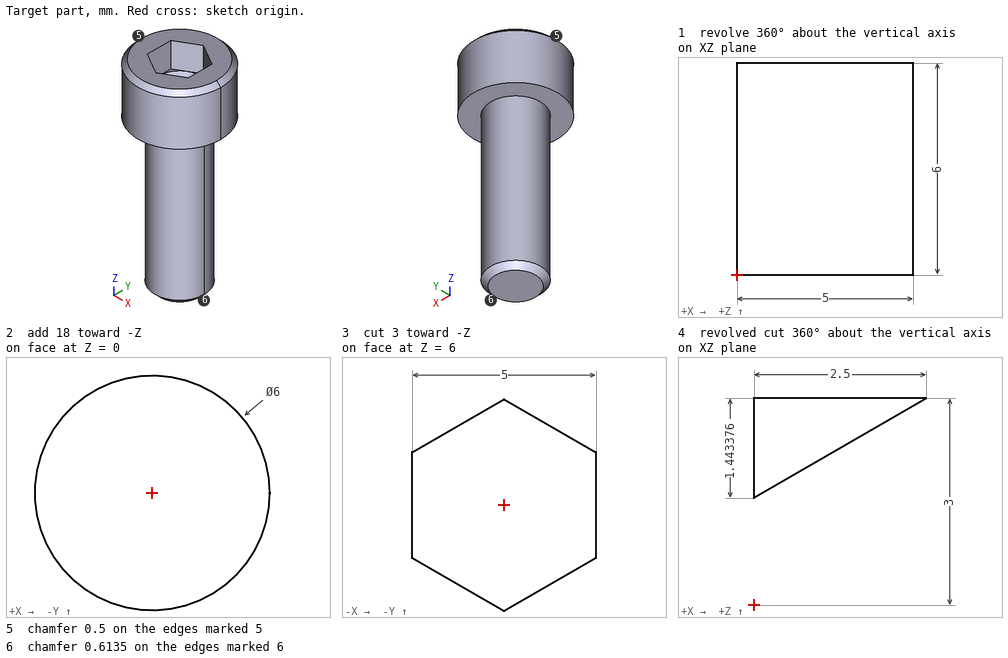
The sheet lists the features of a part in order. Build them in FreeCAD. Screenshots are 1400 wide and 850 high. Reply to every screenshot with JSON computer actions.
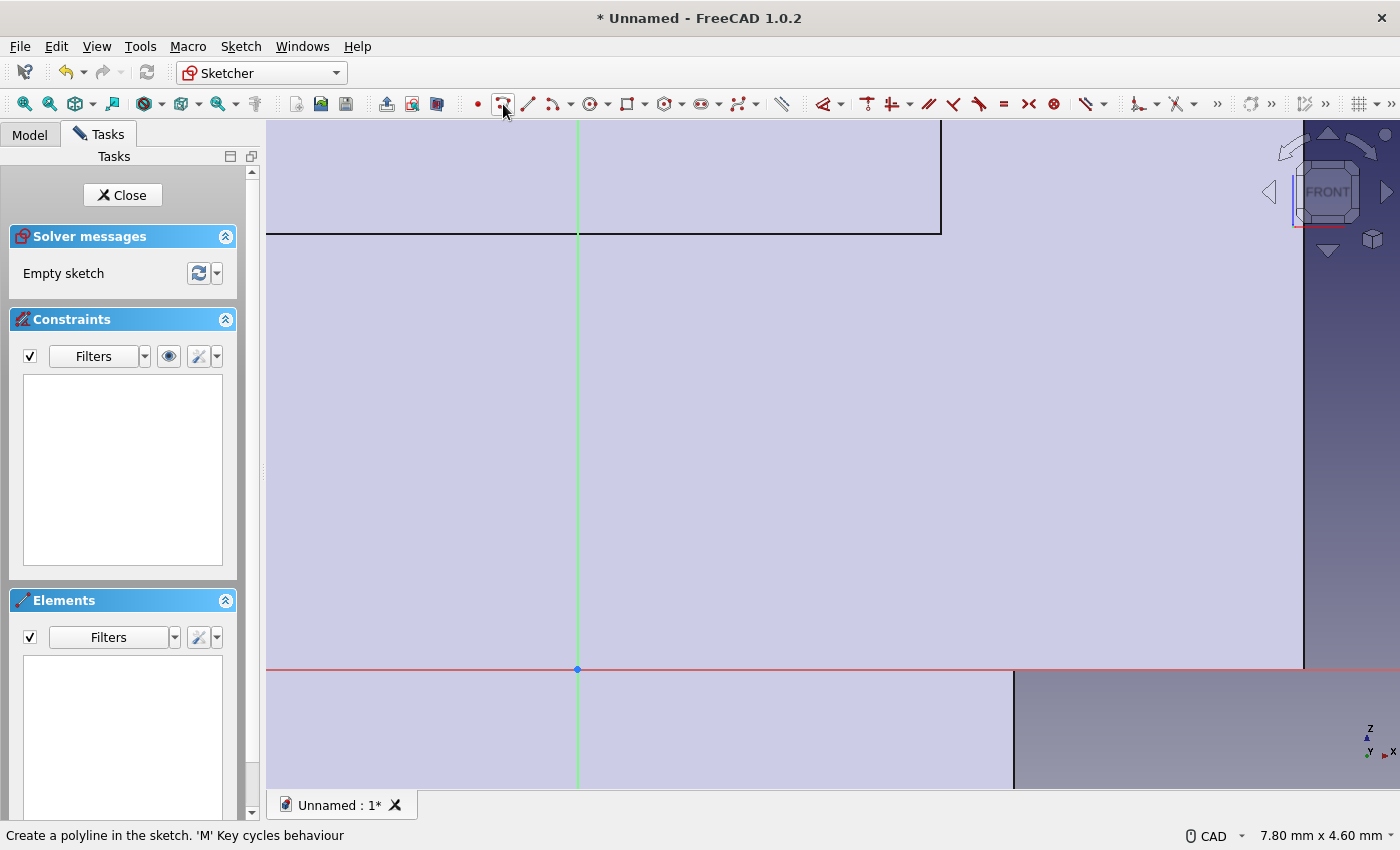
{"action": "left_click", "coordinate": [578, 444]}
{"action": "left_click", "coordinate": [941, 234]}
{"action": "left_click", "coordinate": [587, 234]}
{"action": "left_click", "coordinate": [578, 445]}
{"action": "key", "text": "Escape"}
{"action": "key", "text": "Escape"}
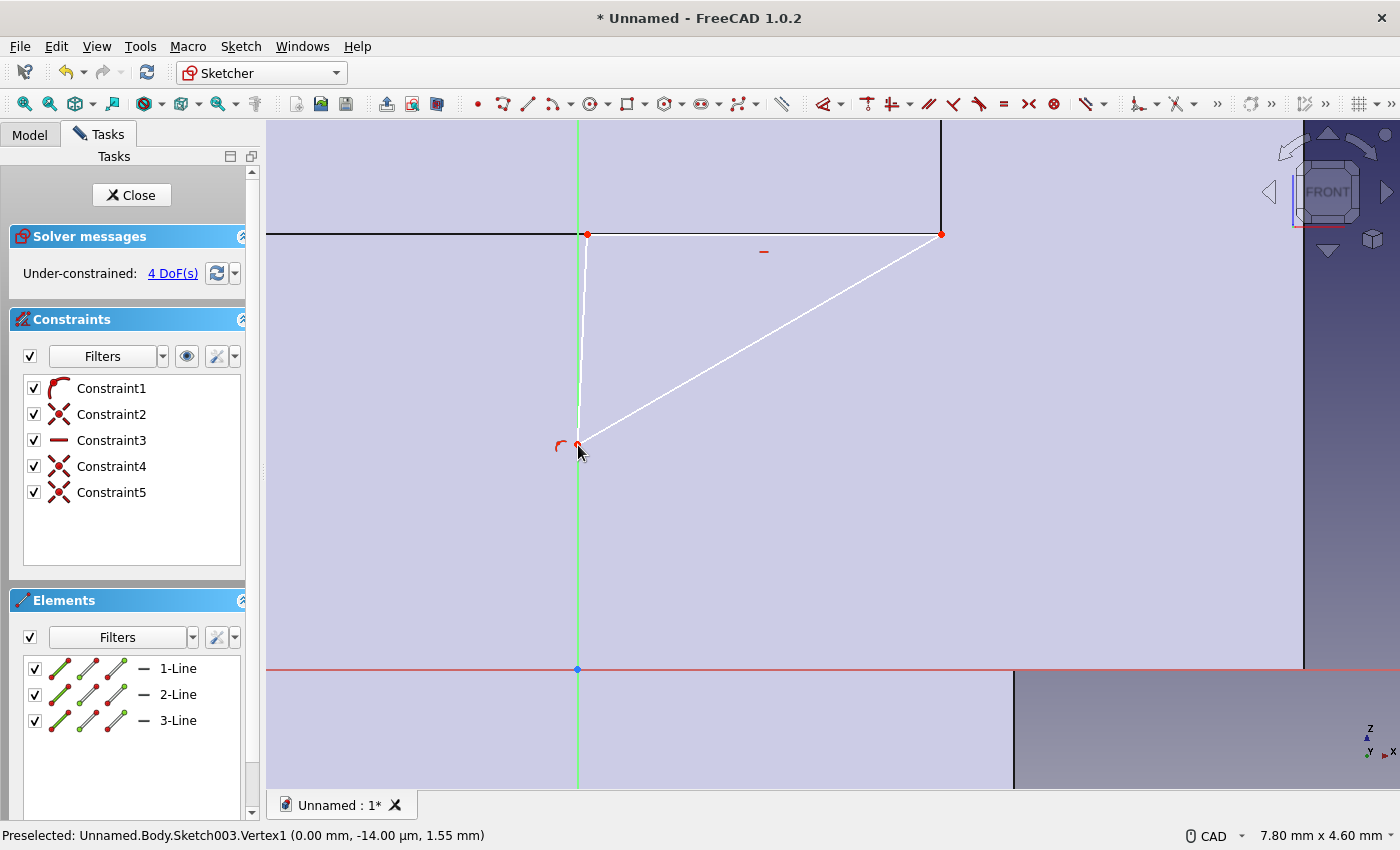
{"action": "left_click", "coordinate": [581, 382]}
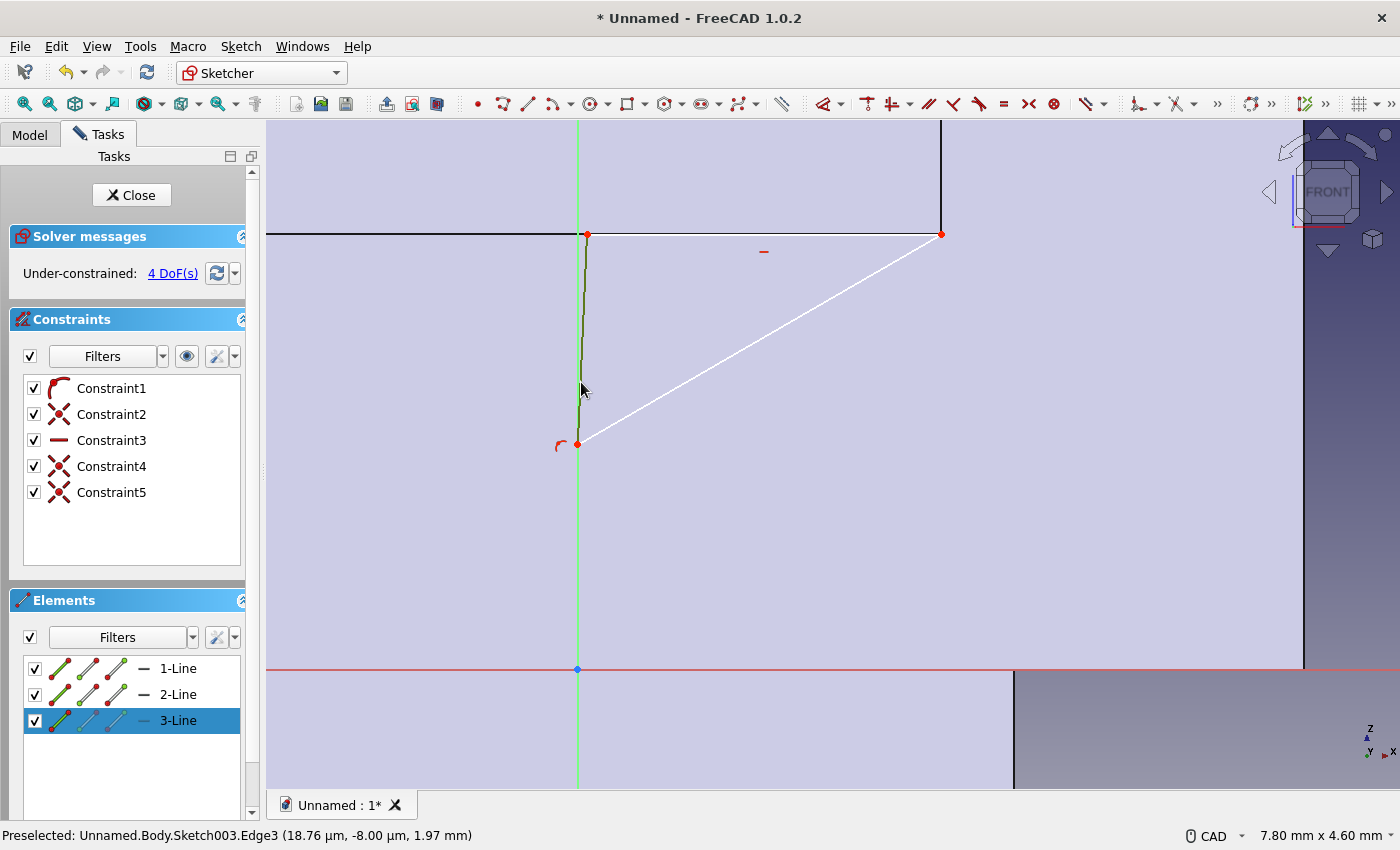
{"action": "left_click", "coordinate": [910, 104]}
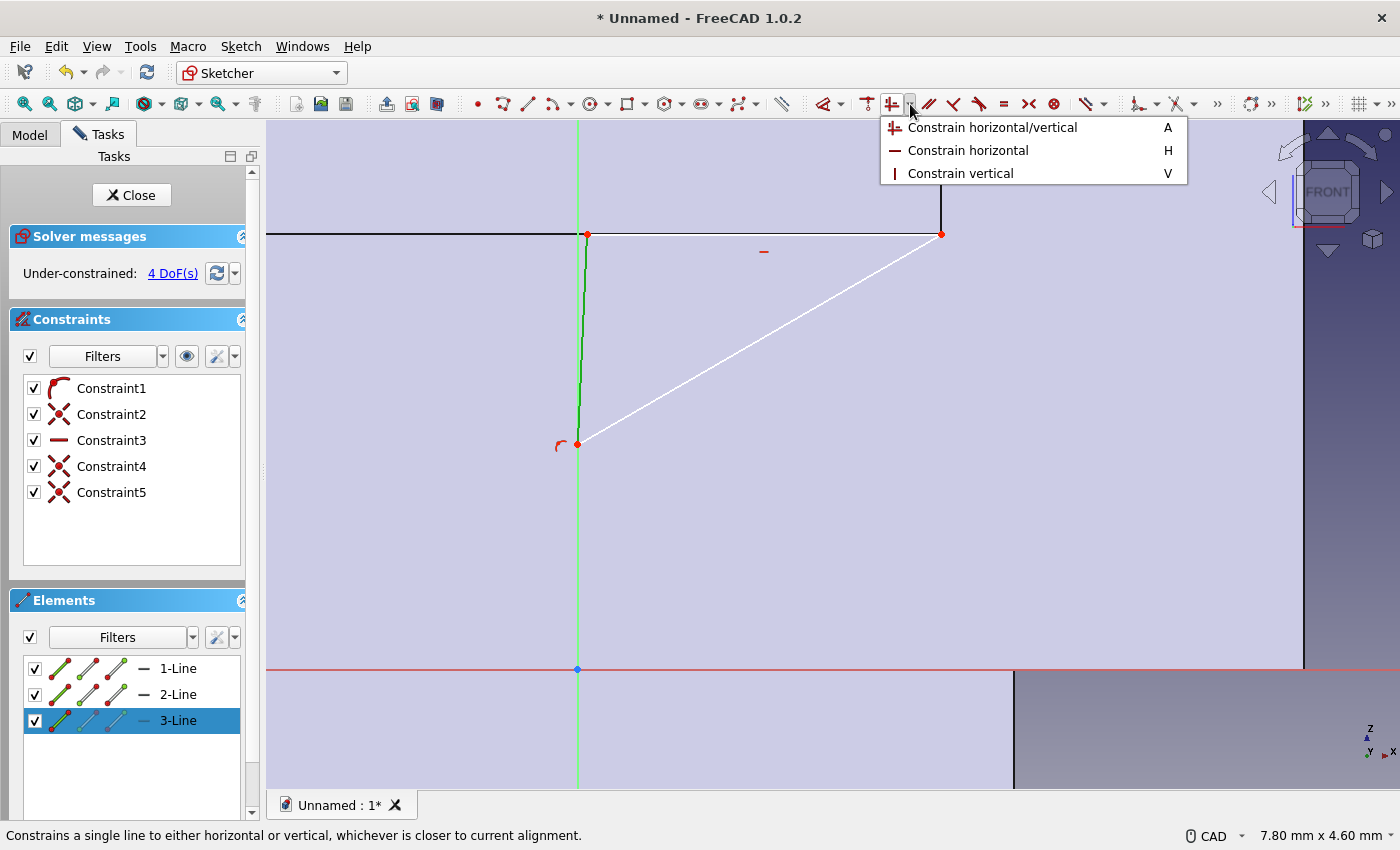
{"action": "left_click", "coordinate": [1034, 174]}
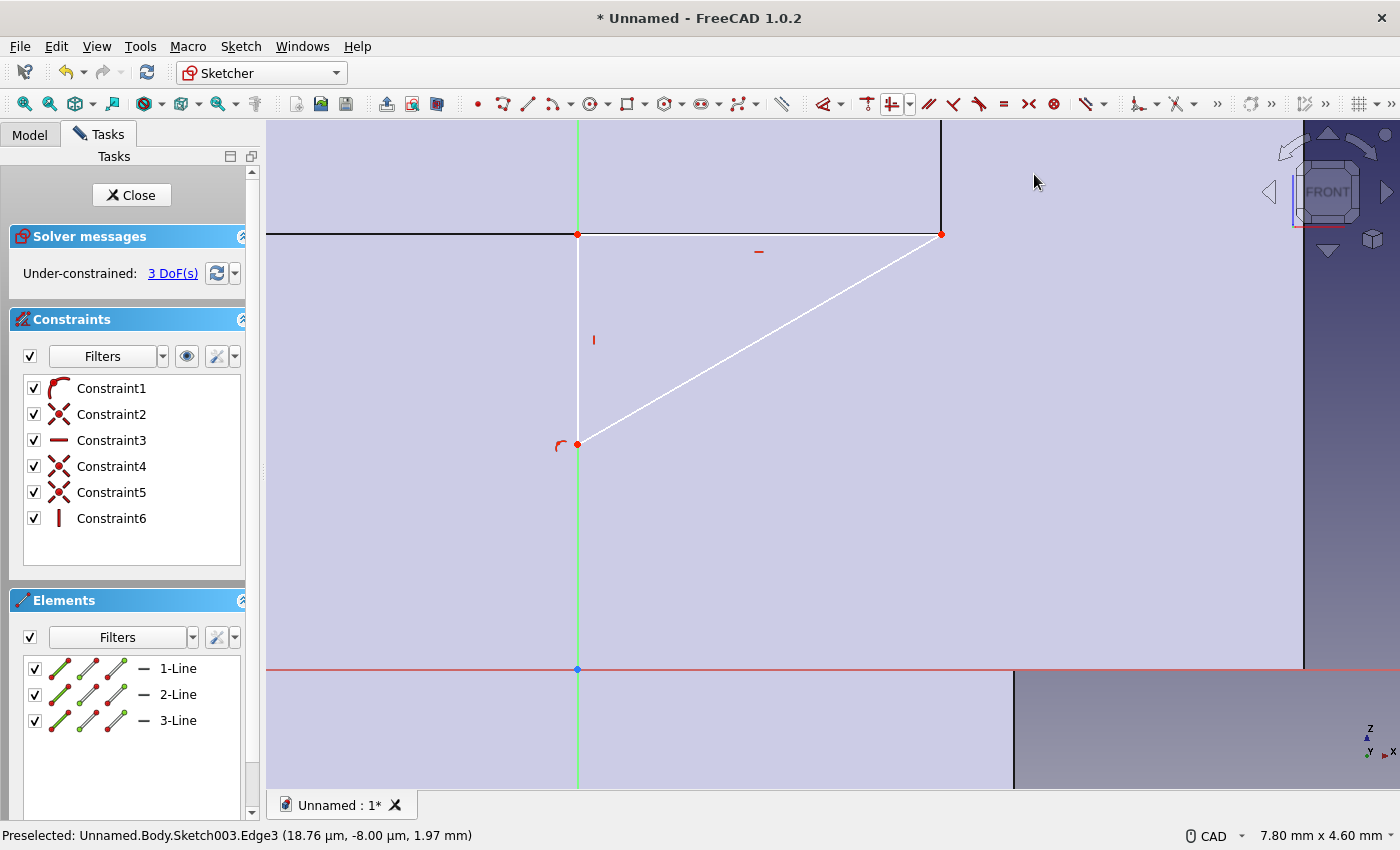
{"action": "left_click", "coordinate": [822, 104]}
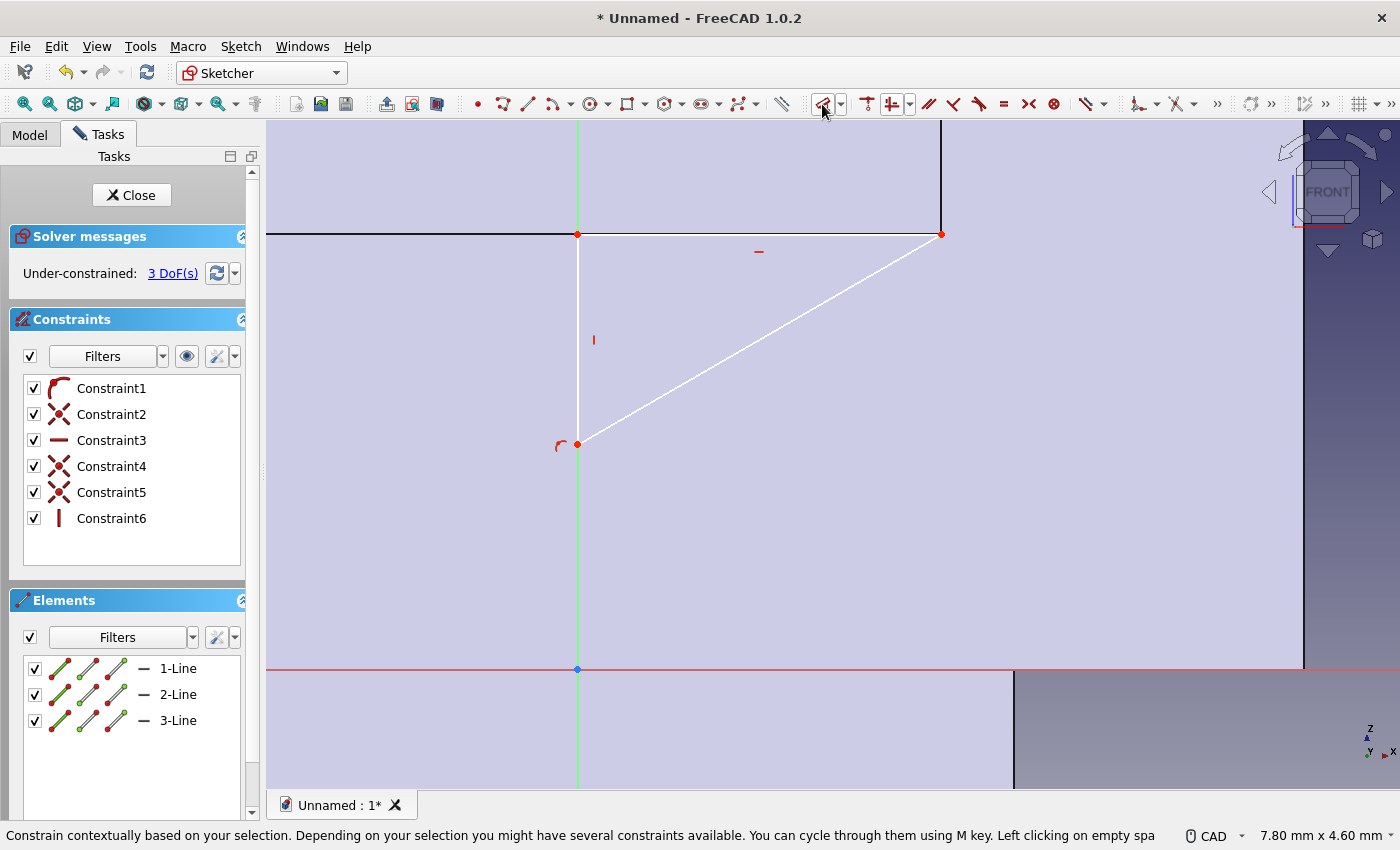
{"action": "left_click", "coordinate": [941, 235]}
{"action": "left_click", "coordinate": [544, 452]}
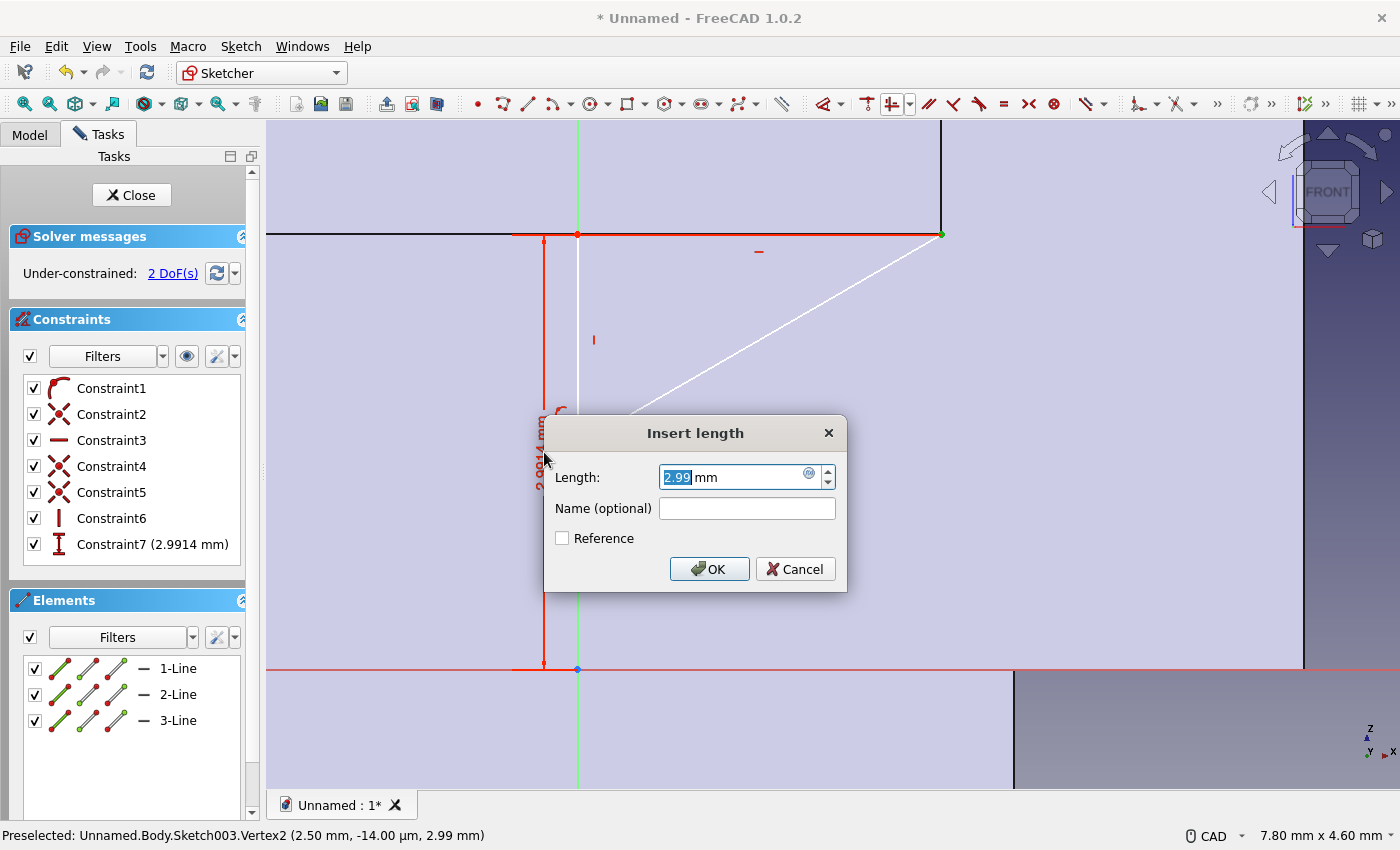
{"action": "type", "text": "3"}
{"action": "key", "text": "Return"}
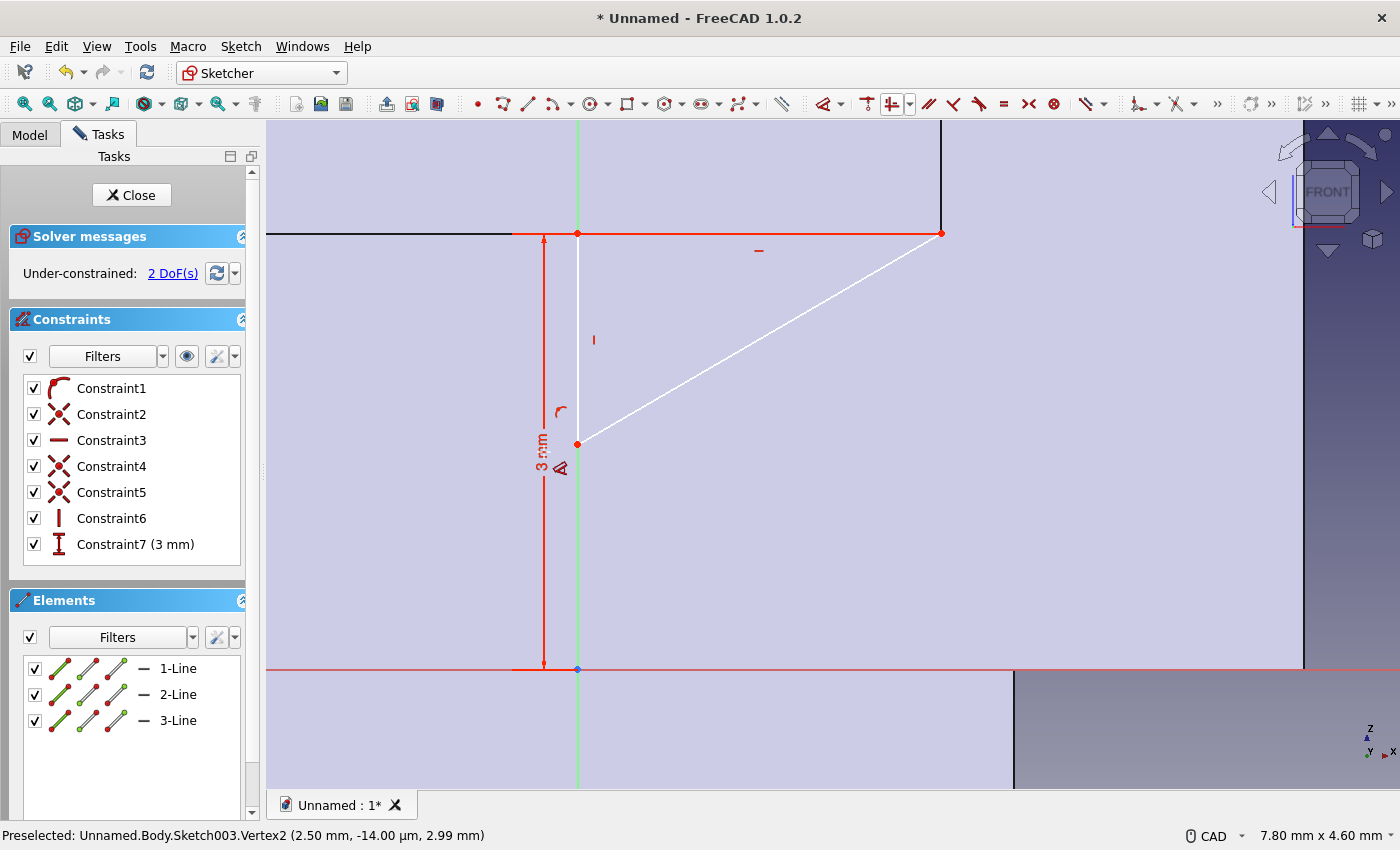
{"action": "left_click", "coordinate": [832, 234]}
{"action": "left_click", "coordinate": [759, 200]}